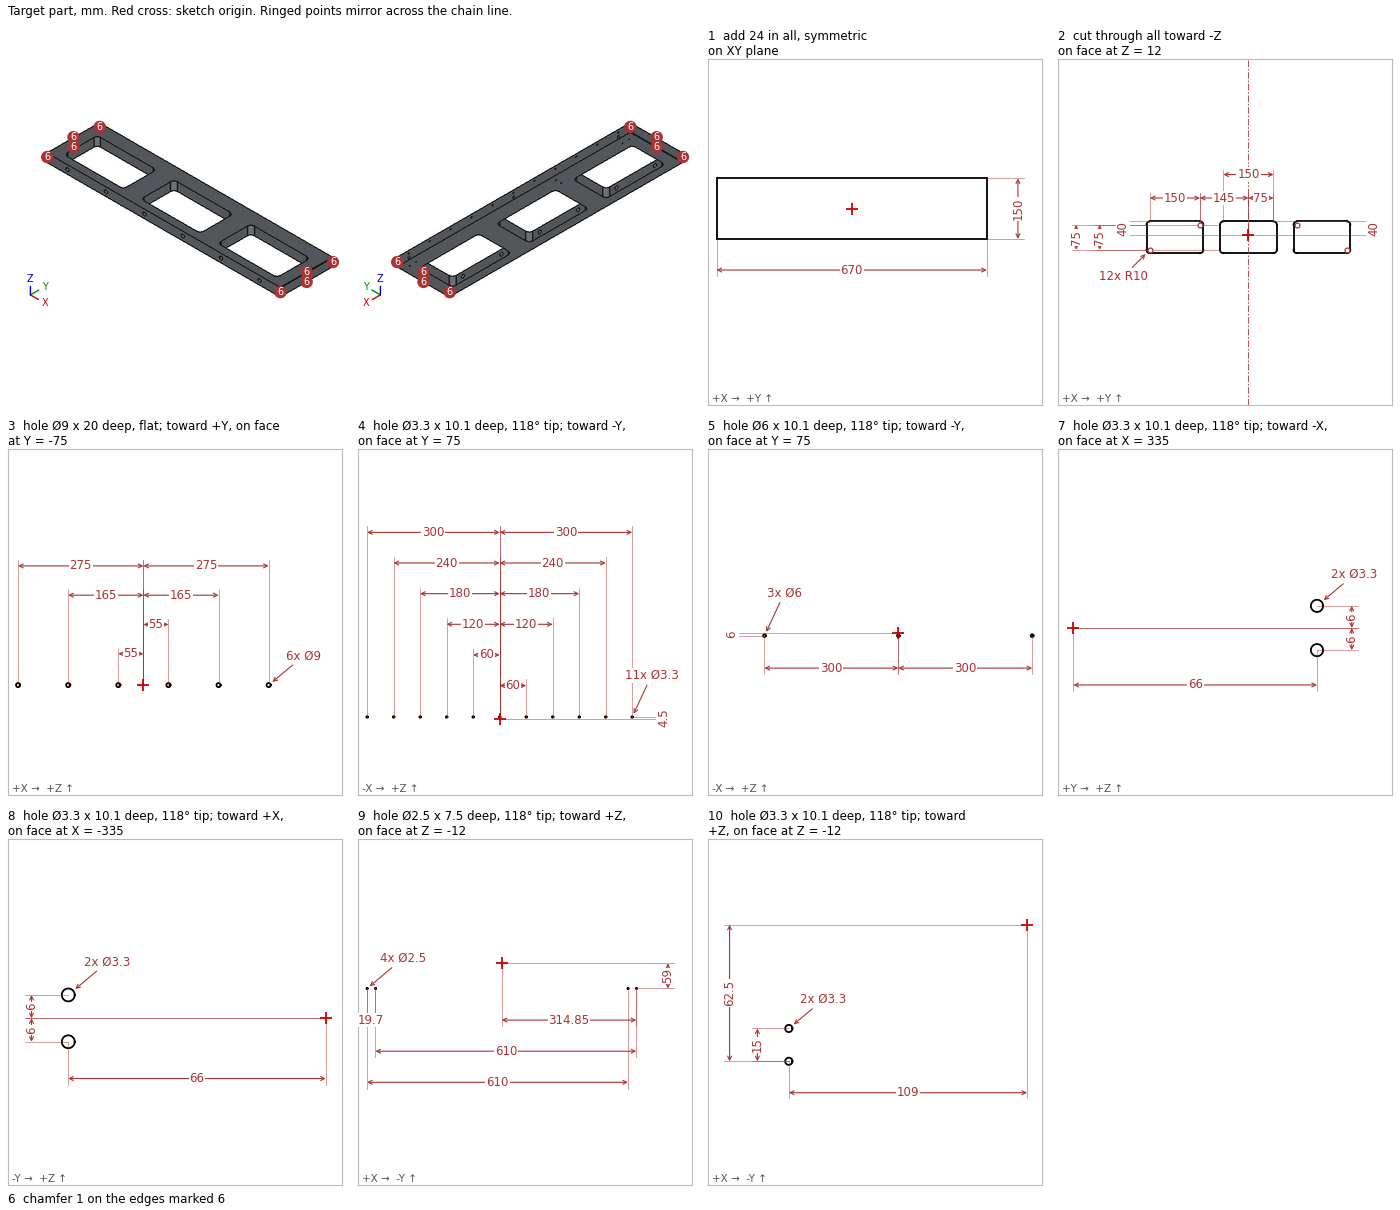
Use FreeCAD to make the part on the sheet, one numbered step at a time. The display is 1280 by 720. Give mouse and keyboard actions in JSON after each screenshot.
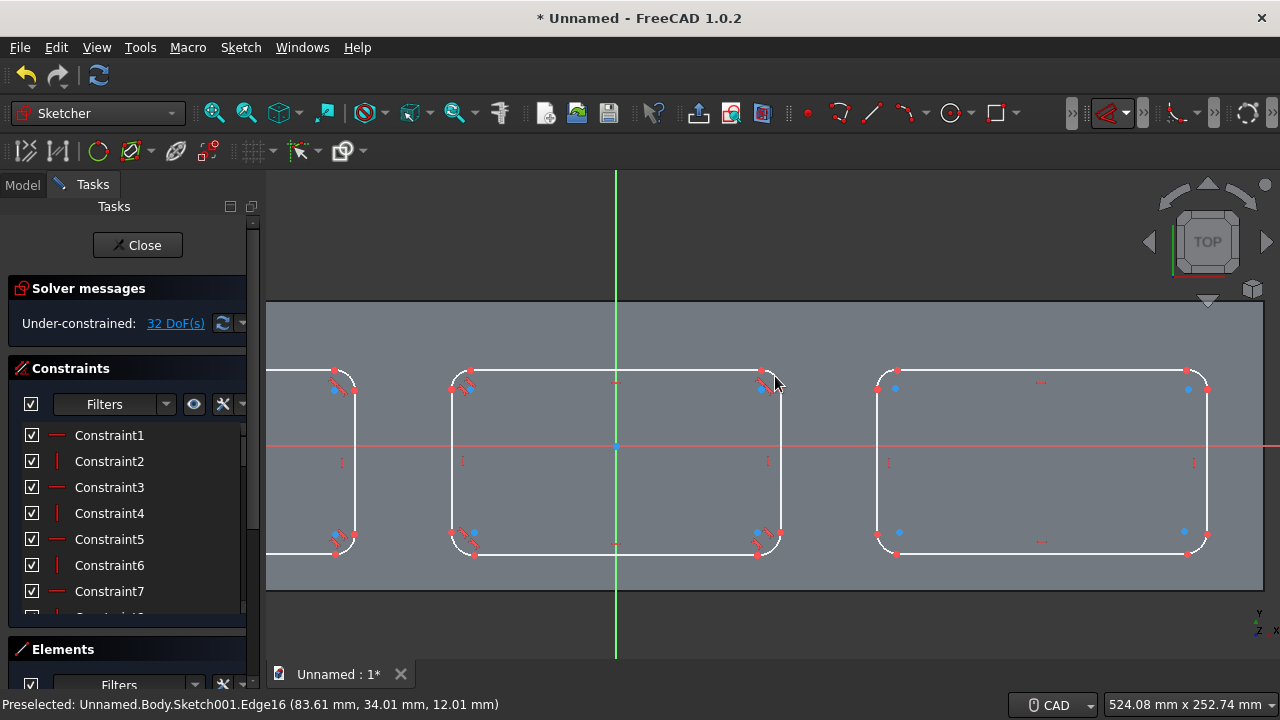
{"action": "left_click", "coordinate": [1100, 370]}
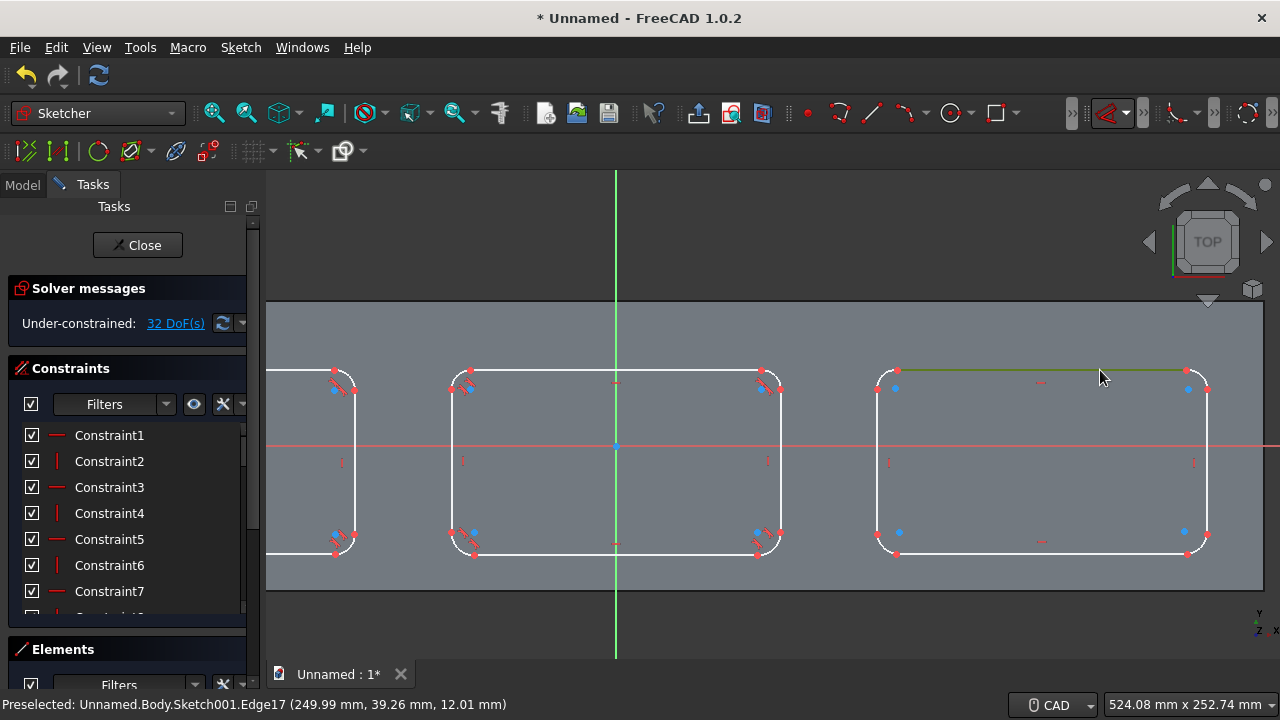
{"action": "scroll", "coordinate": [888, 372], "scroll_direction": "up", "scroll_amount": 2}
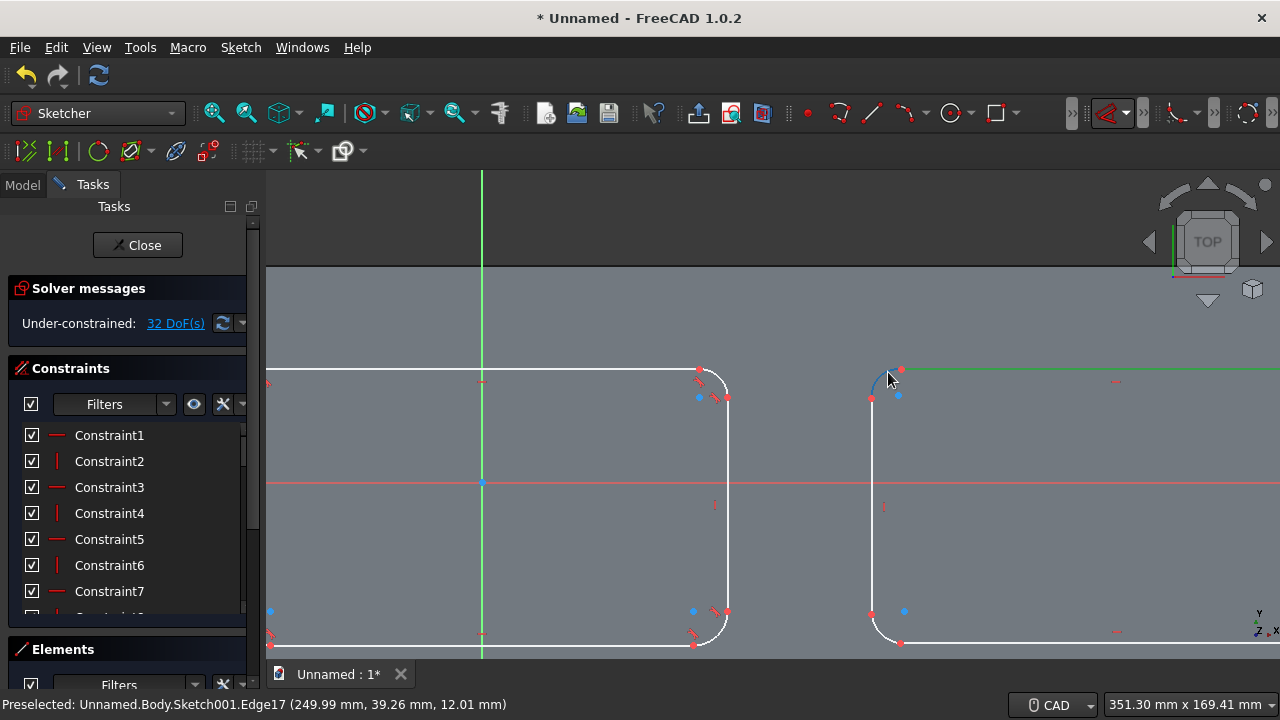
{"action": "left_click", "coordinate": [887, 372]}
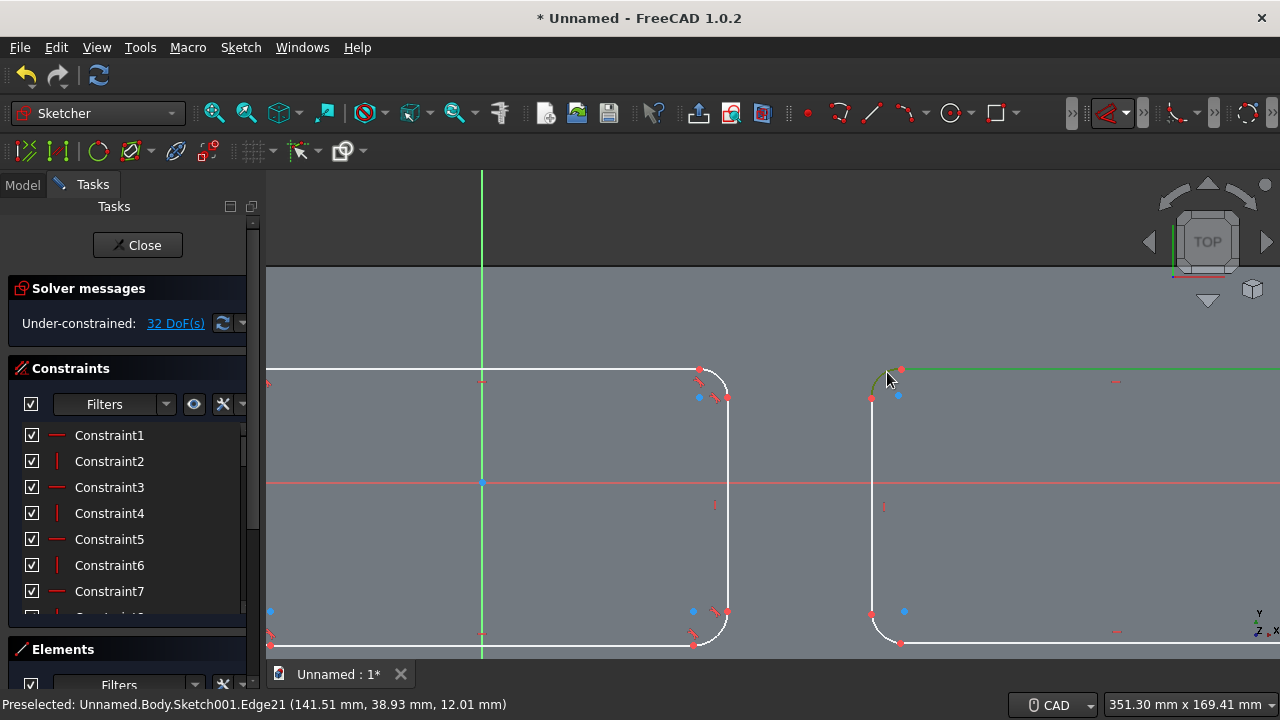
{"action": "key", "text": "t"}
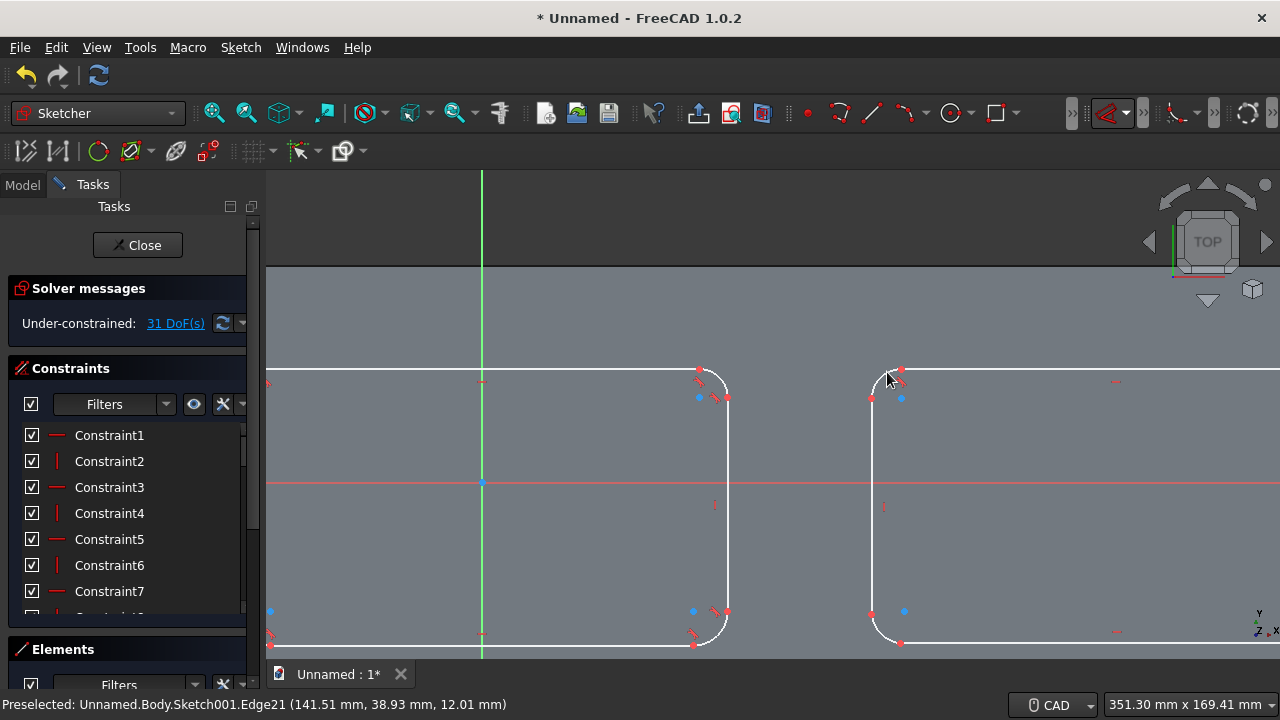
{"action": "scroll", "coordinate": [800, 376], "scroll_direction": "down", "scroll_amount": 6}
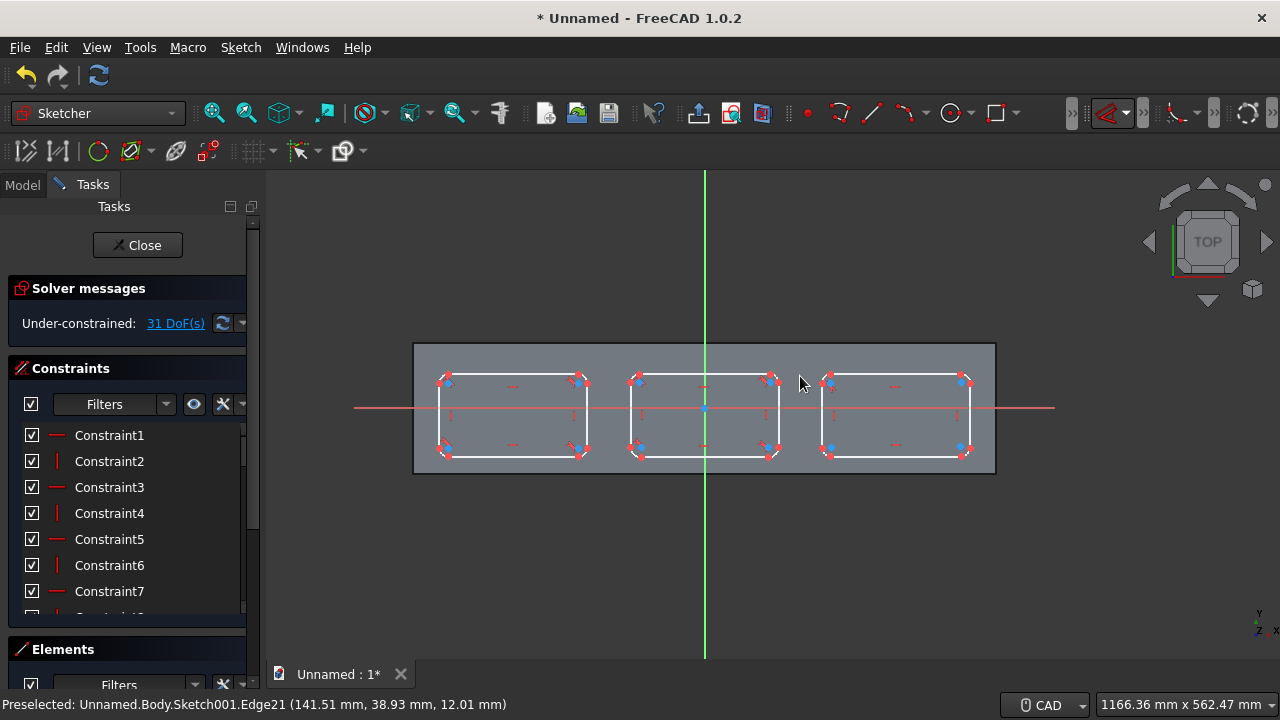
{"action": "left_click", "coordinate": [870, 374]}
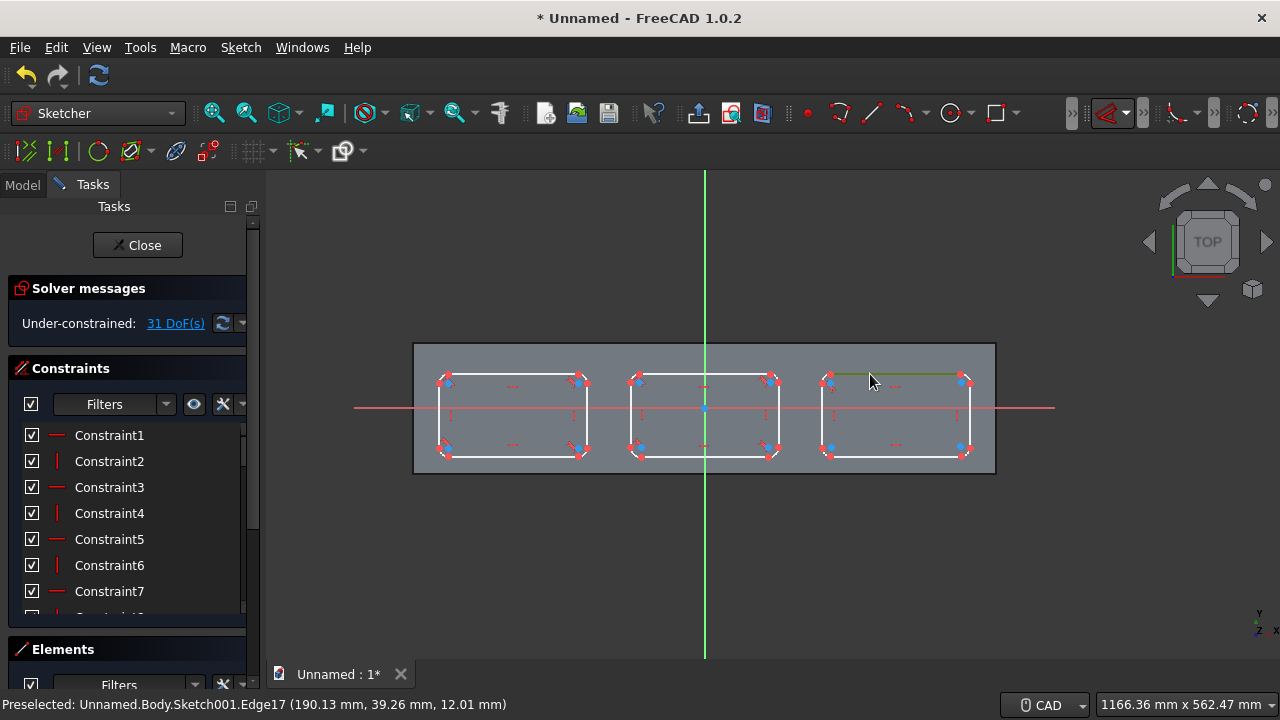
{"action": "scroll", "coordinate": [968, 377], "scroll_direction": "up", "scroll_amount": 4}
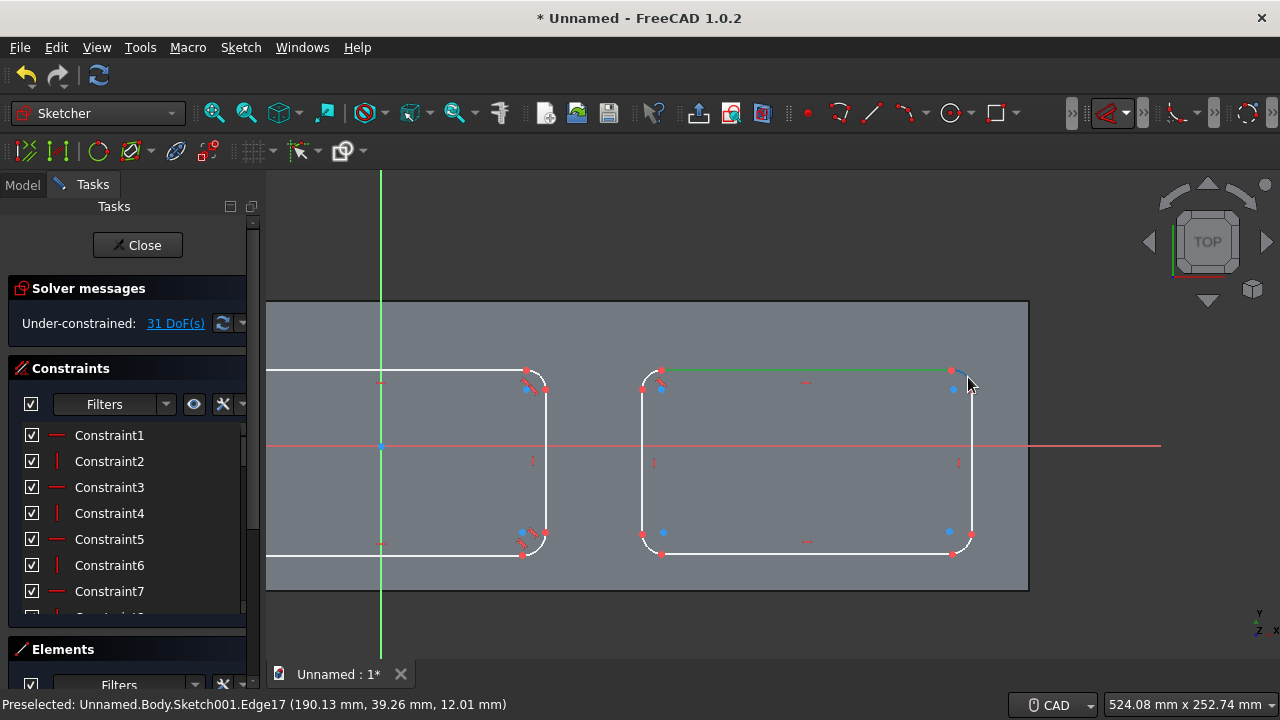
{"action": "left_click", "coordinate": [966, 375]}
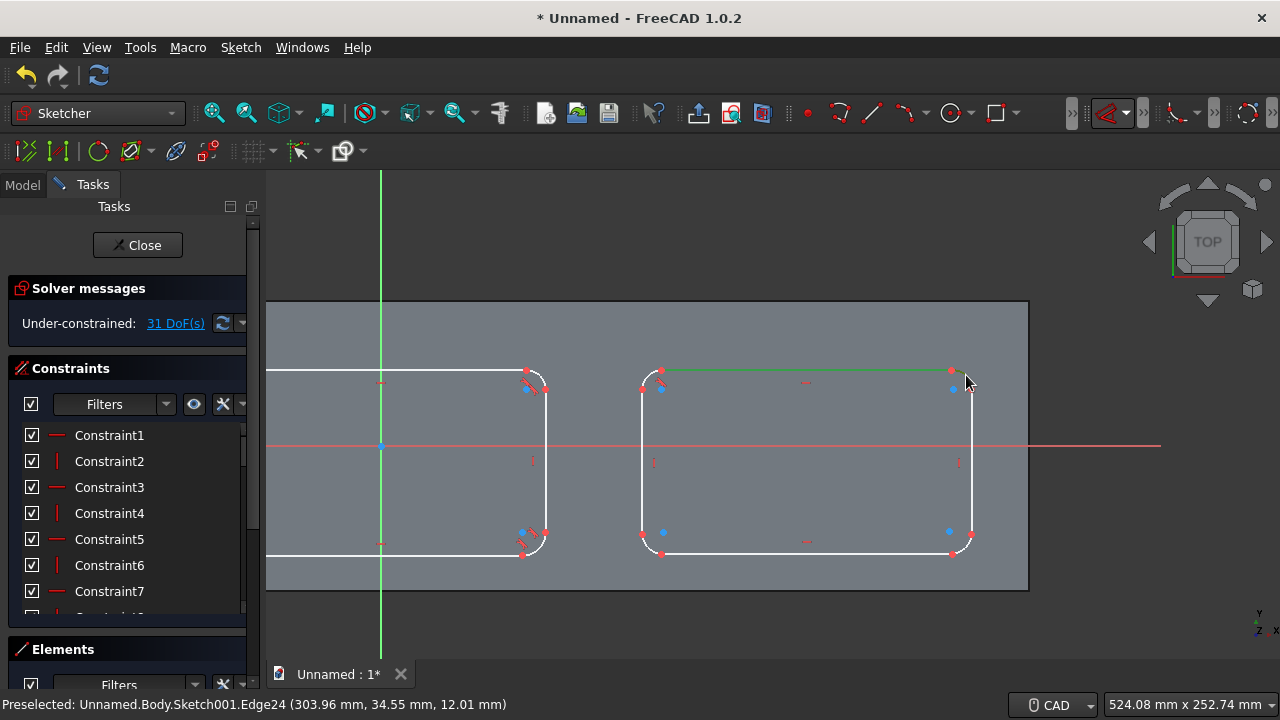
{"action": "key", "text": "t"}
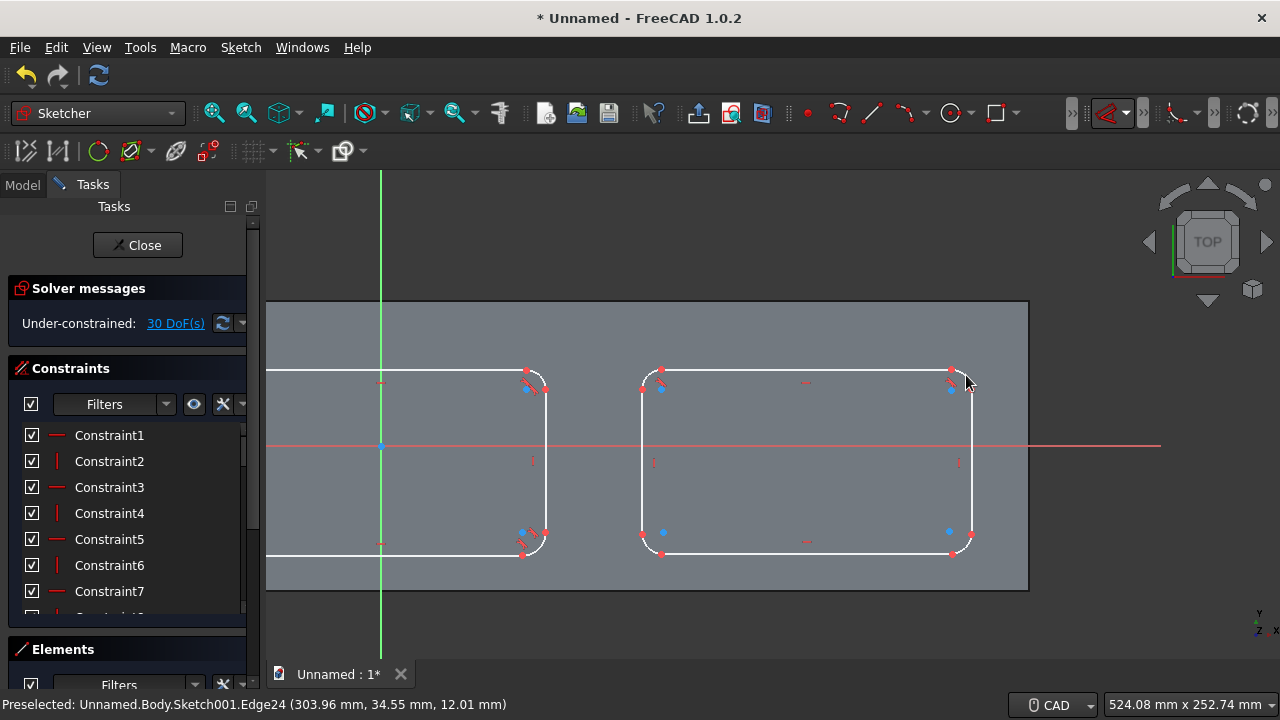
{"action": "left_click", "coordinate": [642, 433]}